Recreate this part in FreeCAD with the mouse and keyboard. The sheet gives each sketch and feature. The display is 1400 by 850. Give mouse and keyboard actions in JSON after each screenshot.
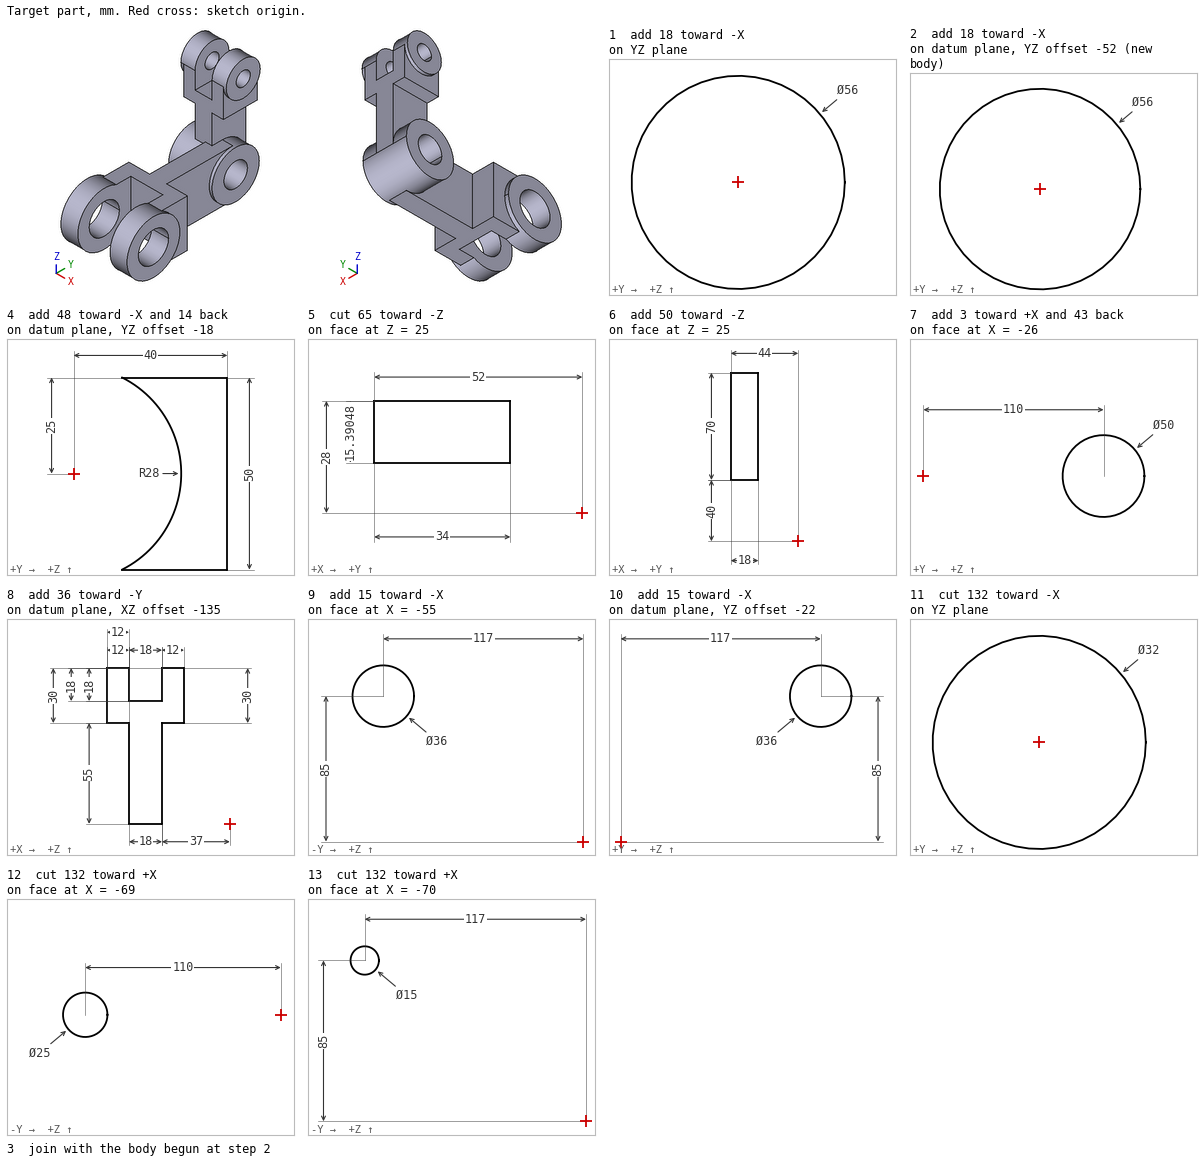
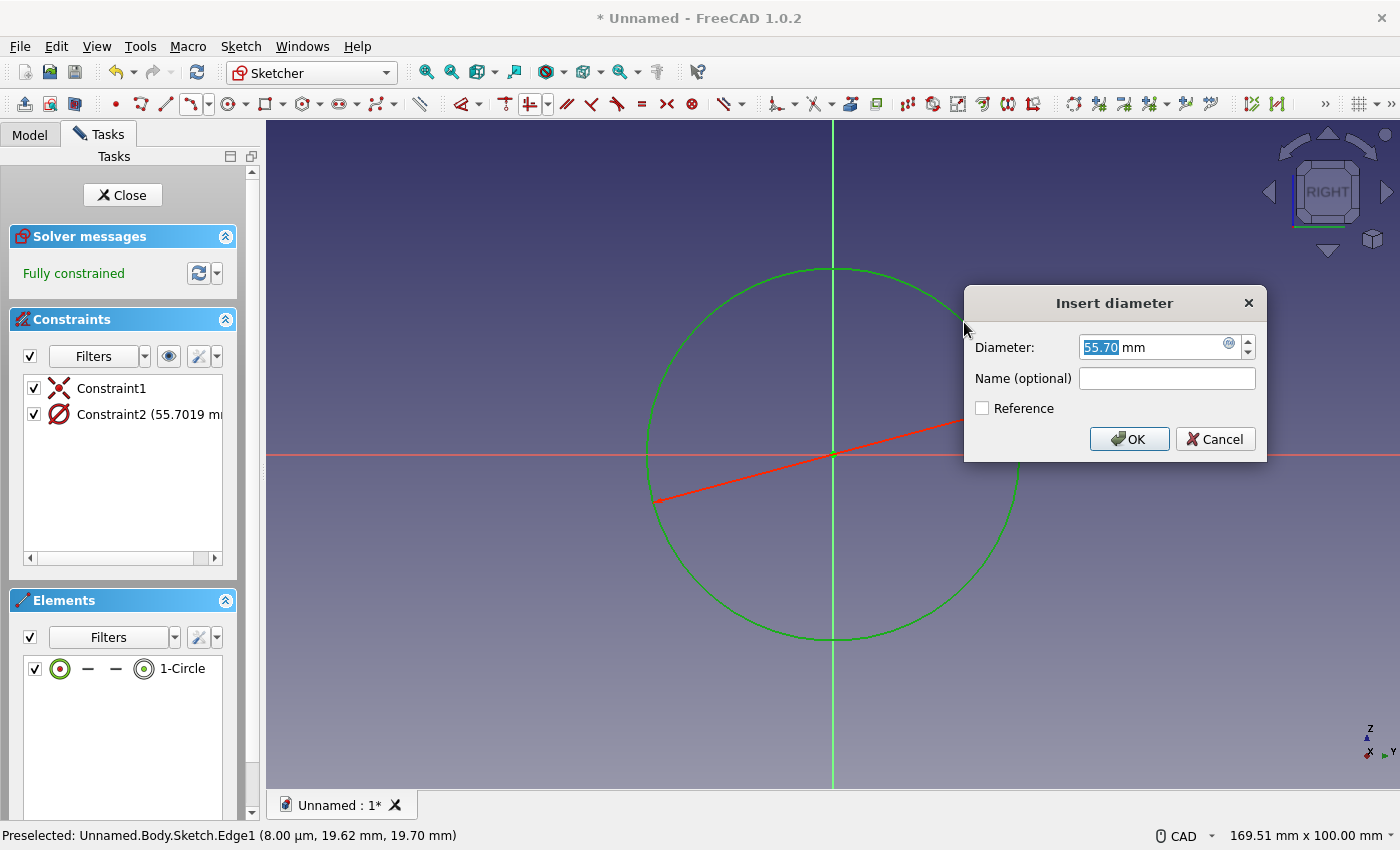
{"action": "type", "text": "56"}
{"action": "key", "text": "Return"}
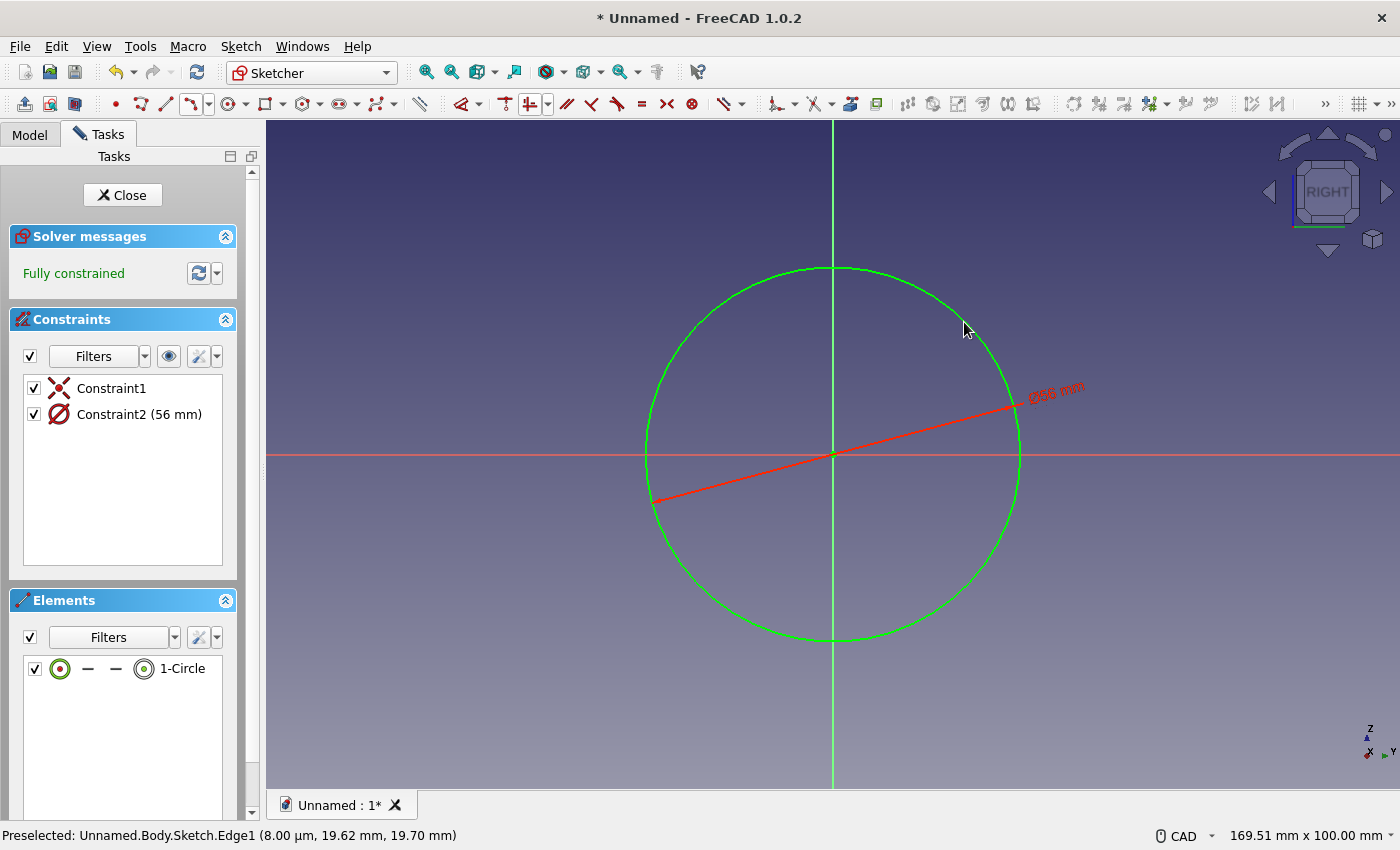
{"action": "left_click", "coordinate": [123, 195]}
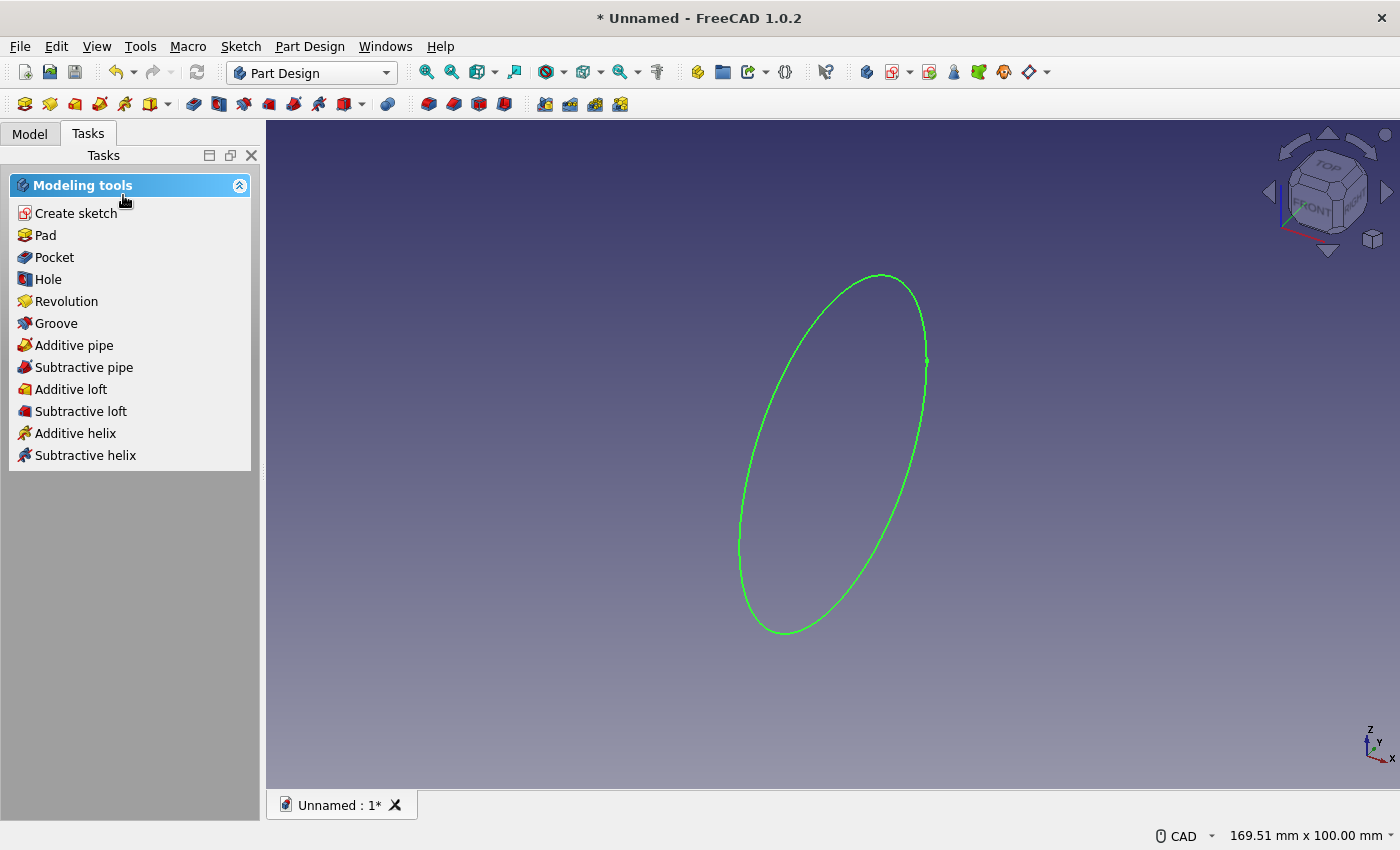
{"action": "left_click", "coordinate": [25, 104]}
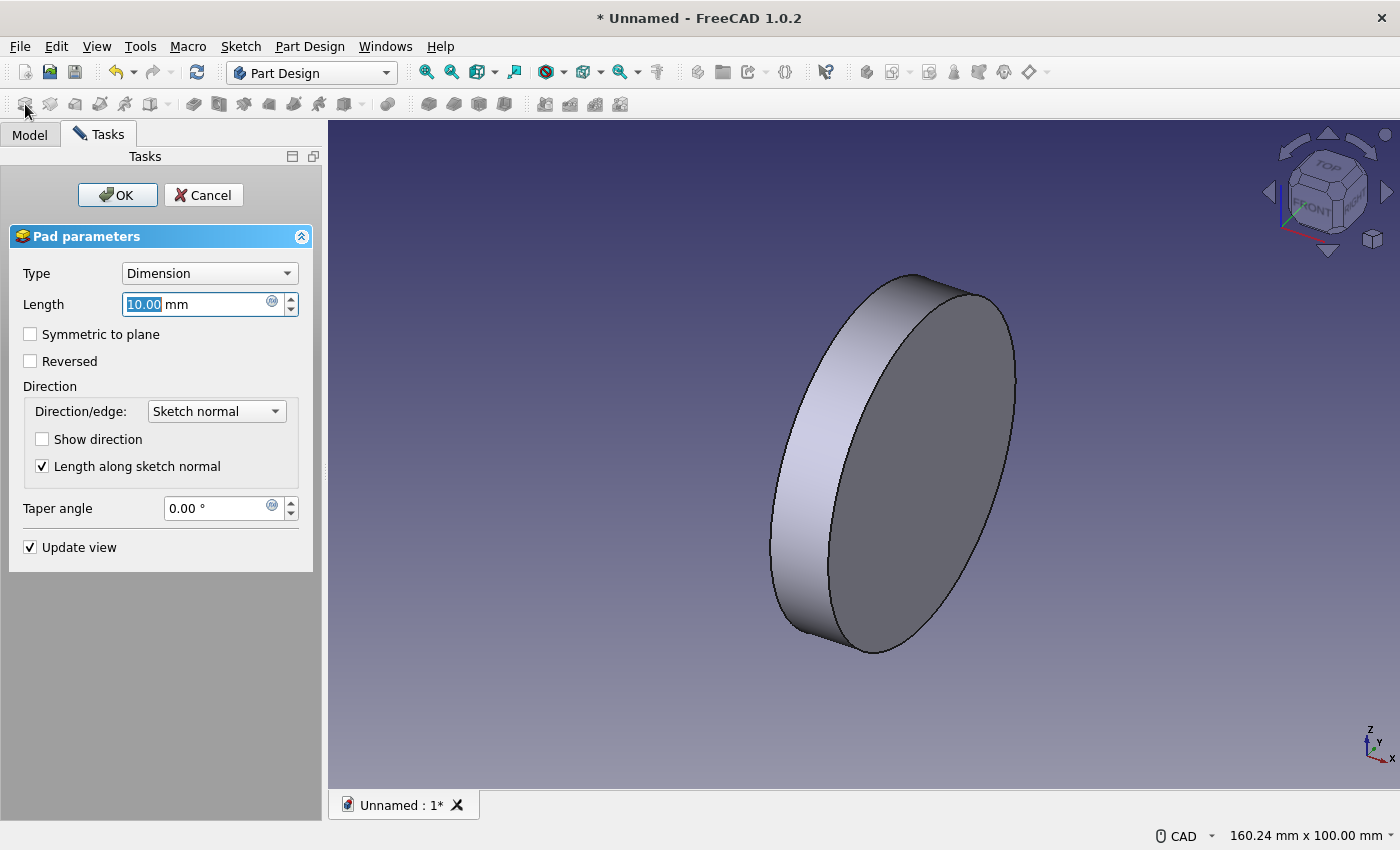
{"action": "type", "text": "18"}
{"action": "key", "text": "Tab"}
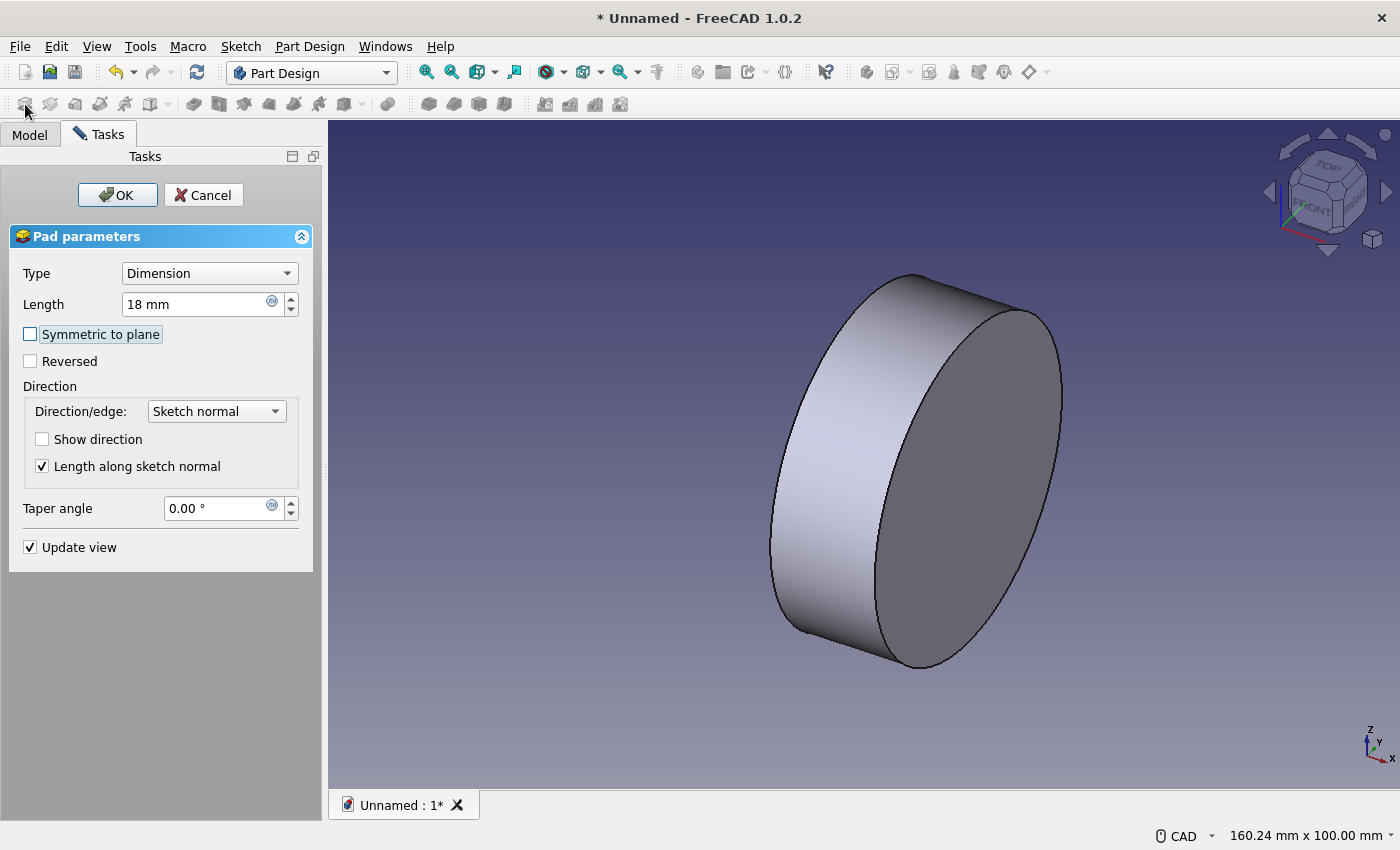
{"action": "left_click", "coordinate": [31, 361]}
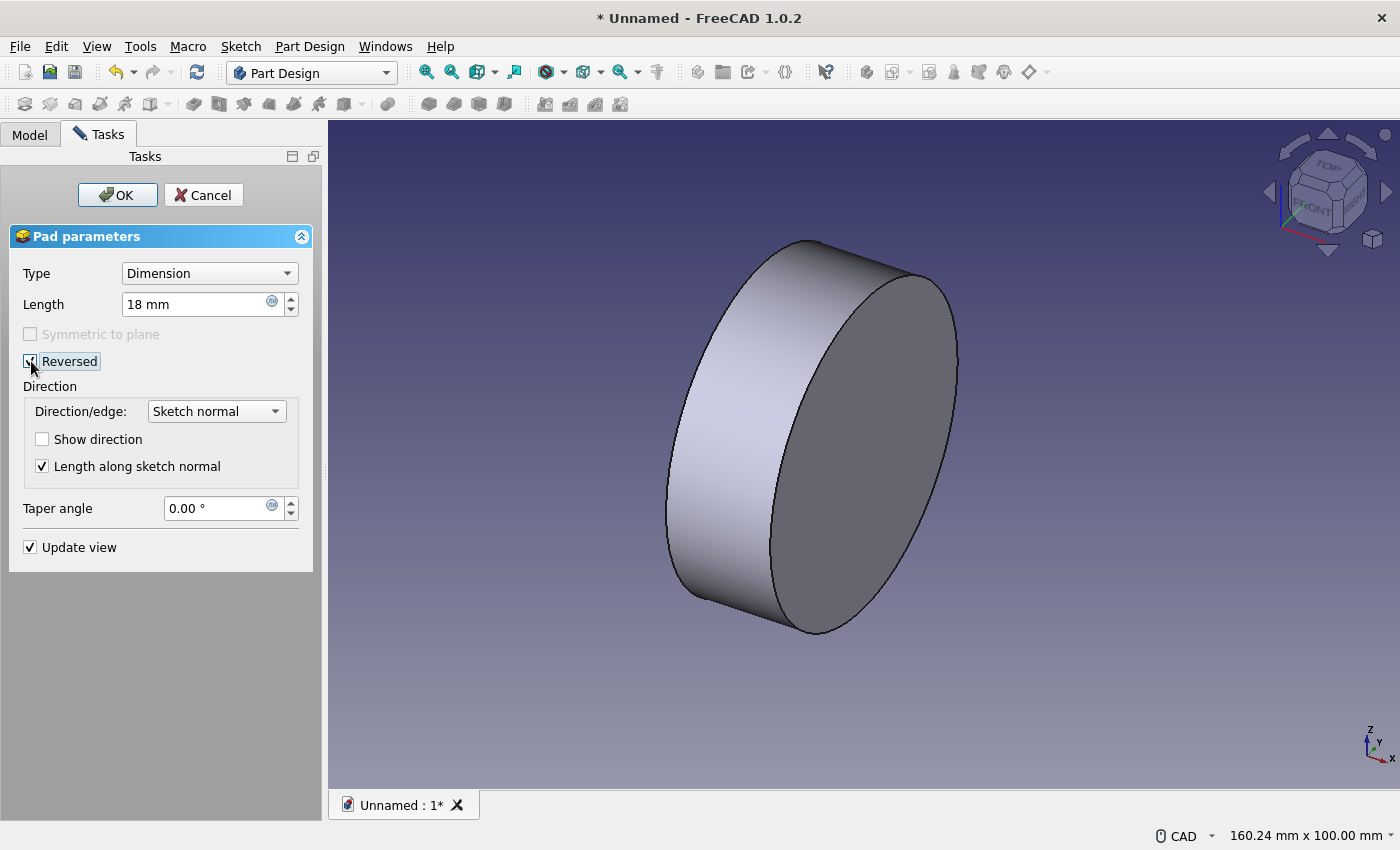
{"action": "left_click", "coordinate": [118, 195]}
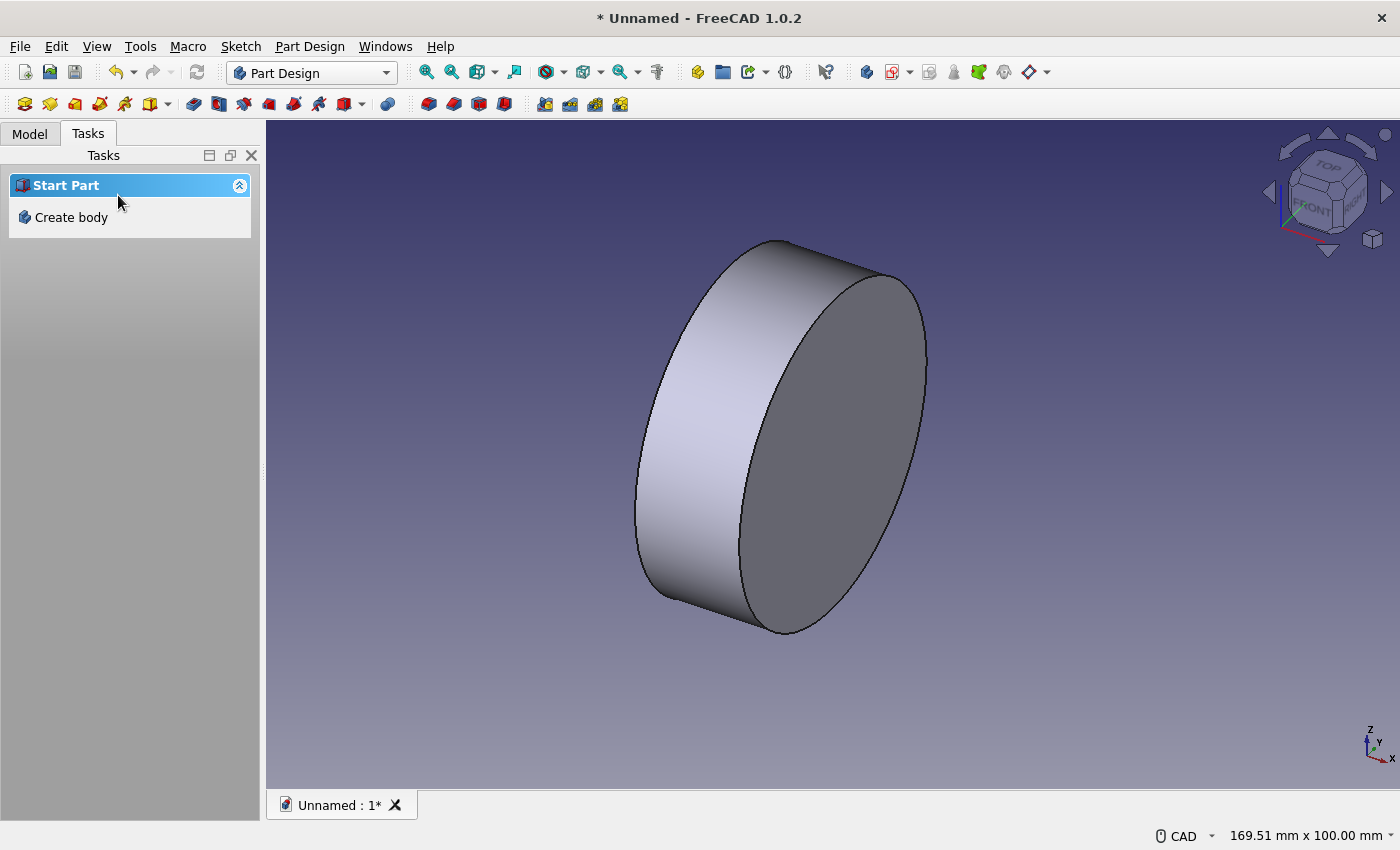
{"action": "left_click", "coordinate": [867, 72]}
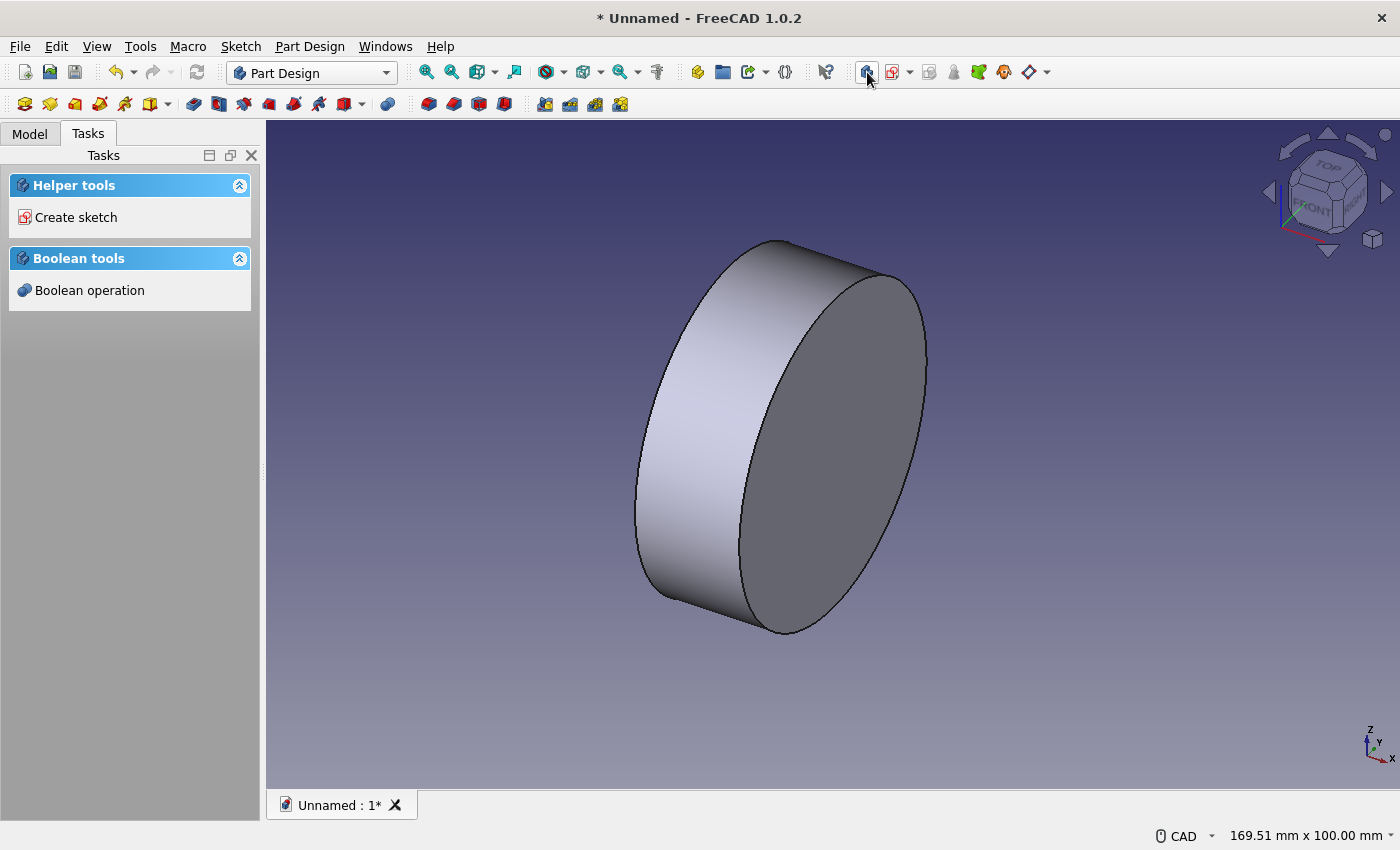
{"action": "left_click", "coordinate": [30, 134]}